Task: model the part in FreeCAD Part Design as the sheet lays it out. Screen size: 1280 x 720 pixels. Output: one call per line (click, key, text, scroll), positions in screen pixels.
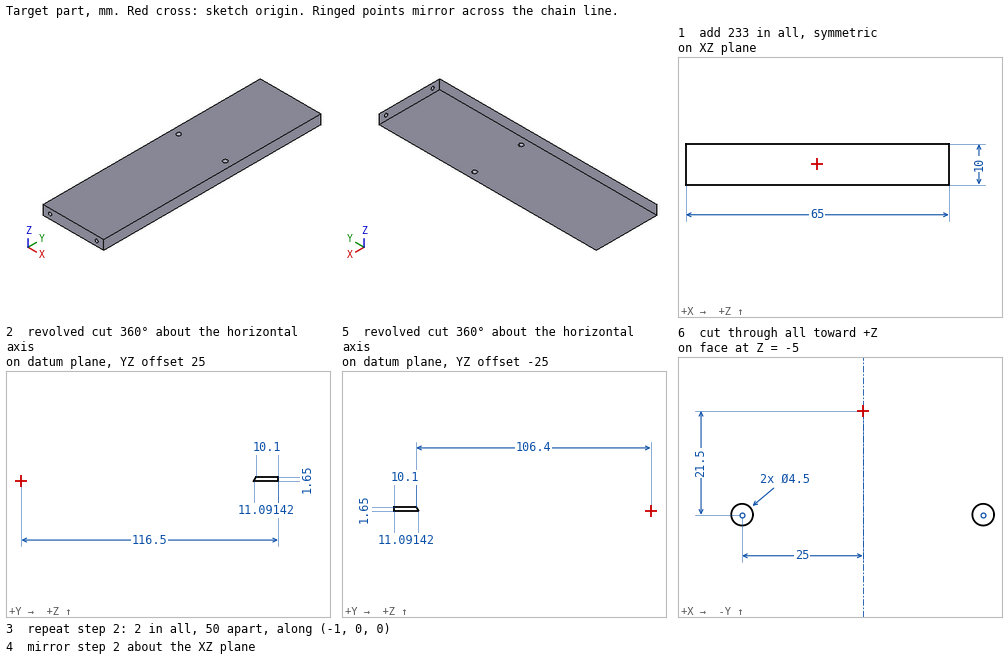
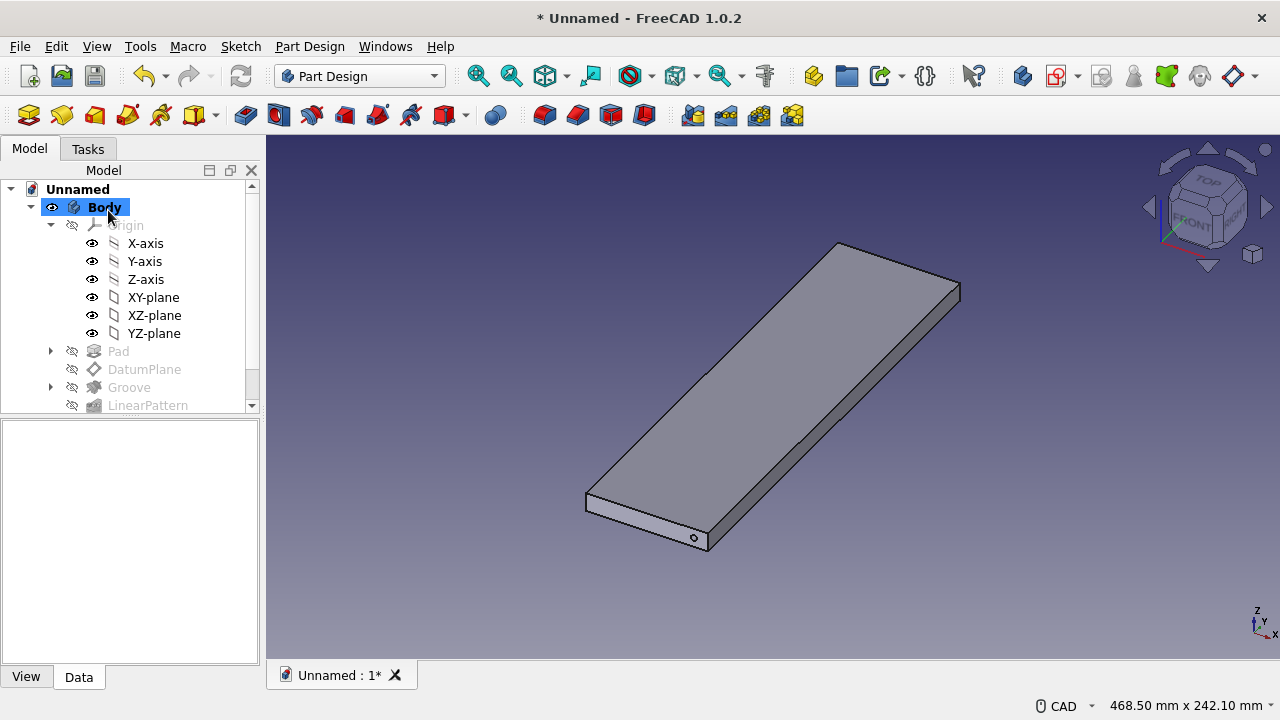
click(137, 333)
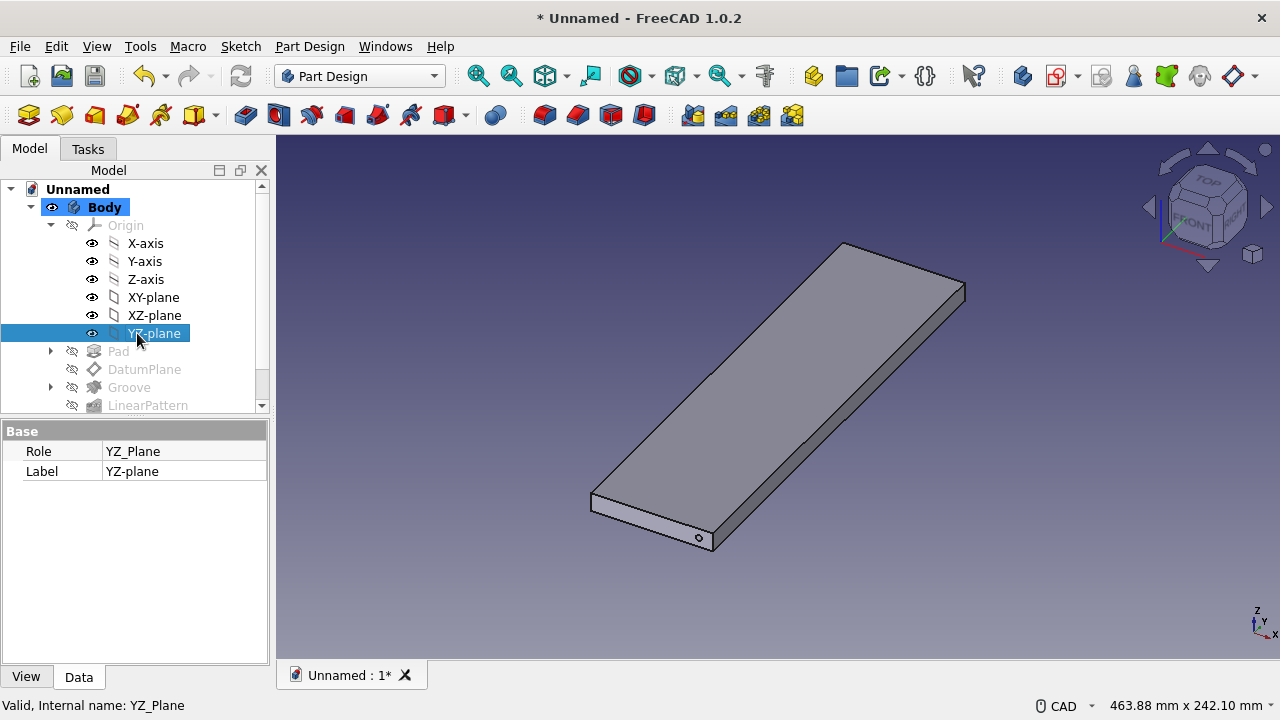
click(1232, 76)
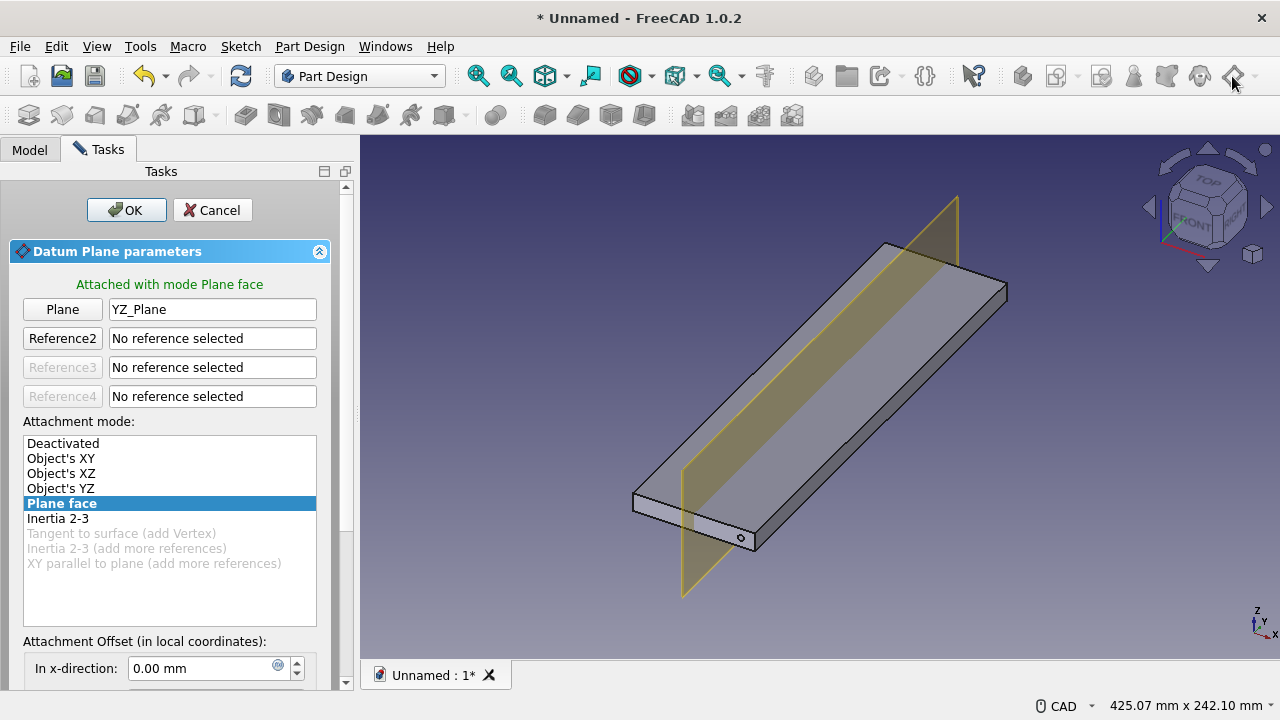
scroll(346, 436, down, 2)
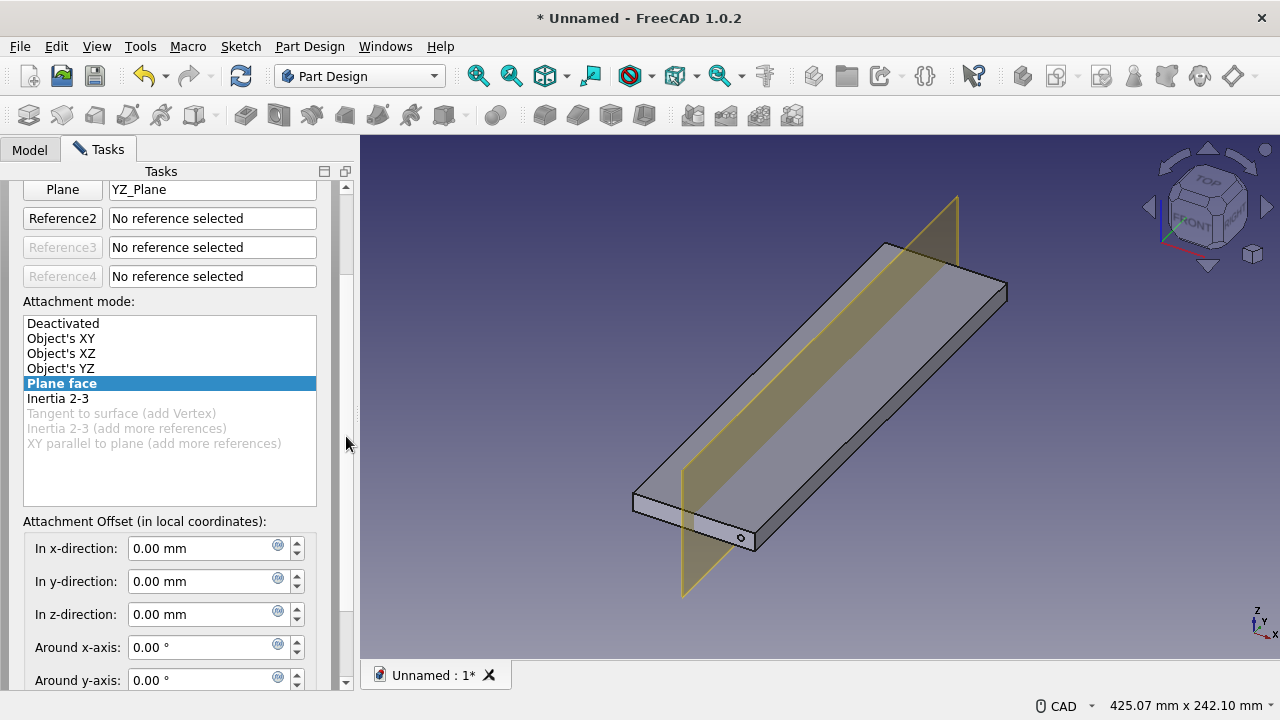
triple_click(210, 614)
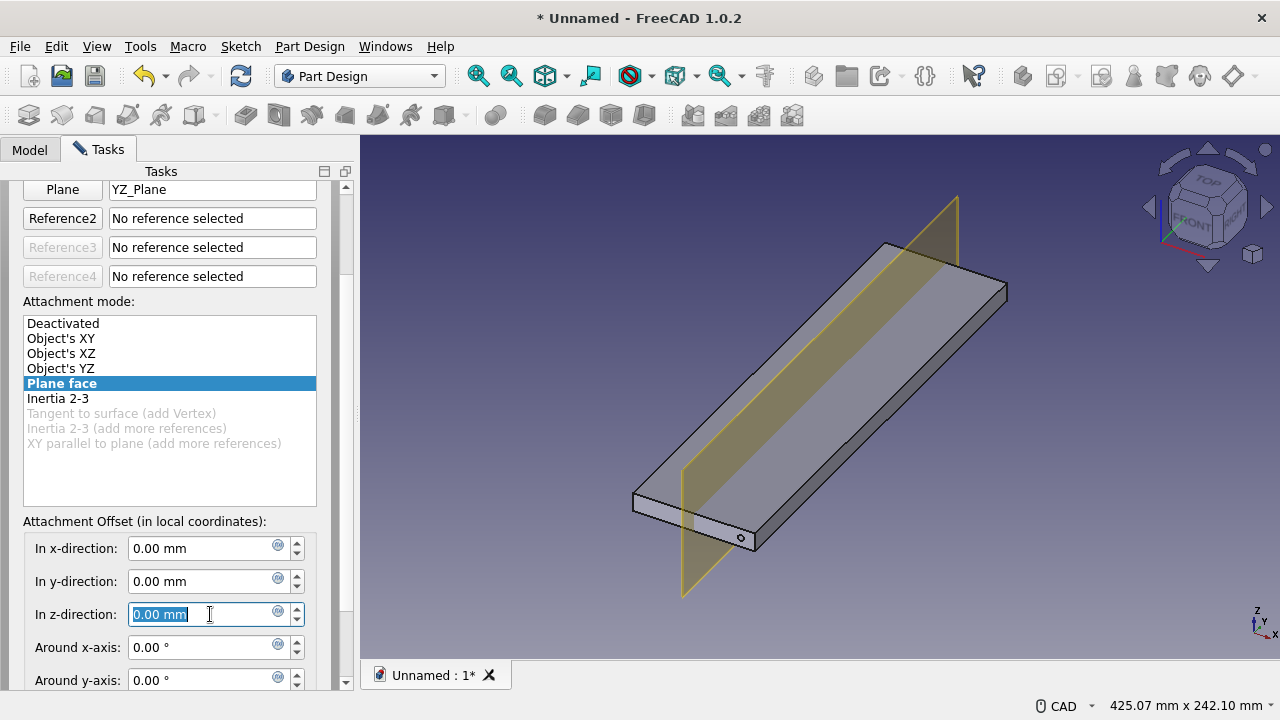
text(-25)
key(Tab)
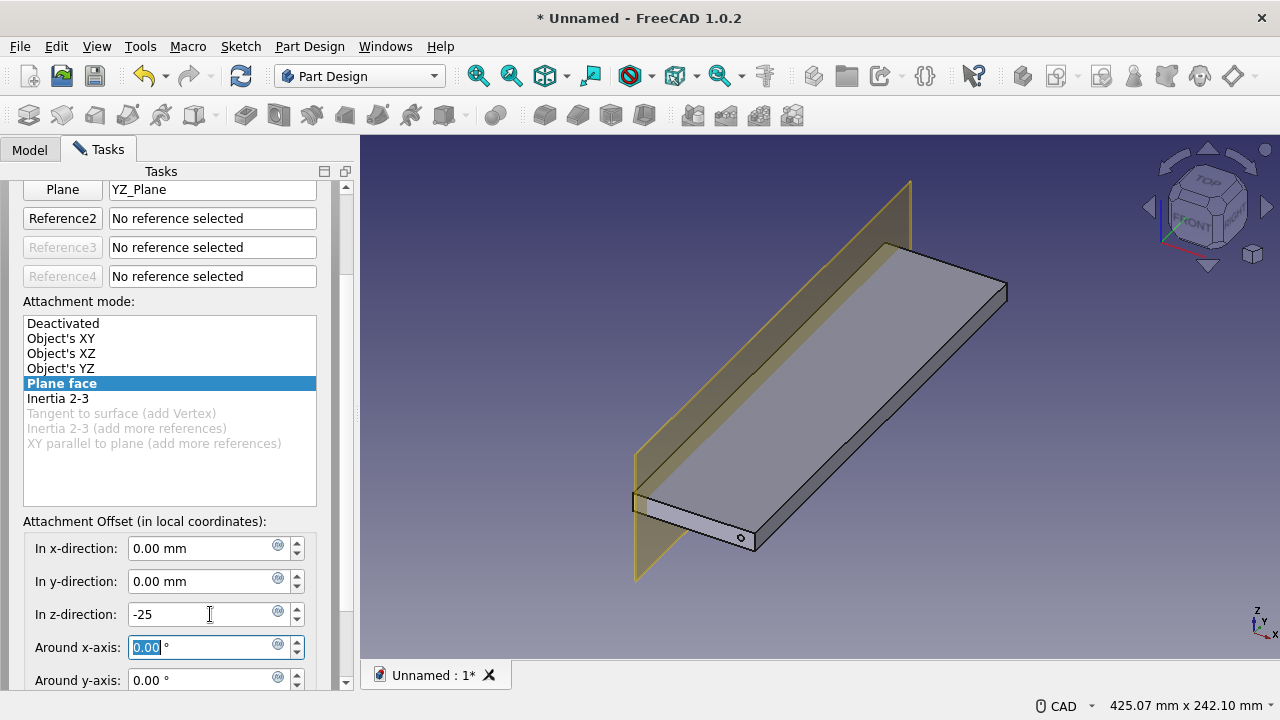
scroll(346, 436, up, 3)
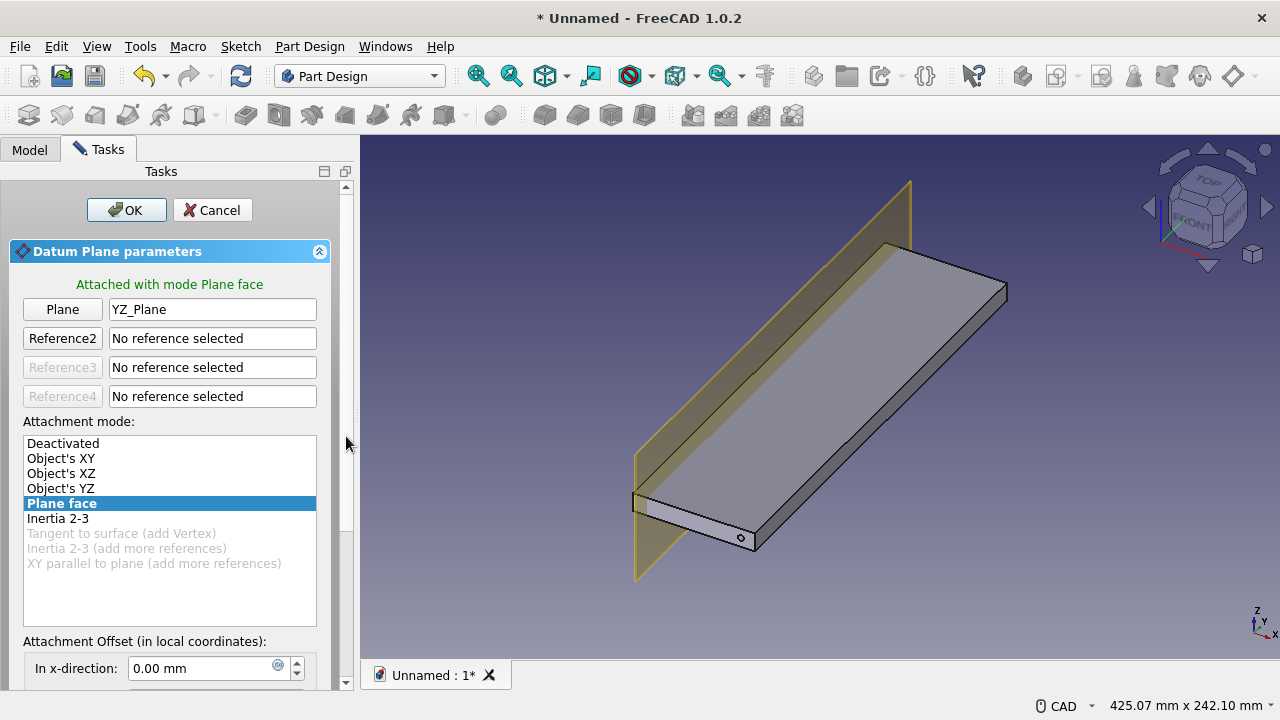
click(127, 210)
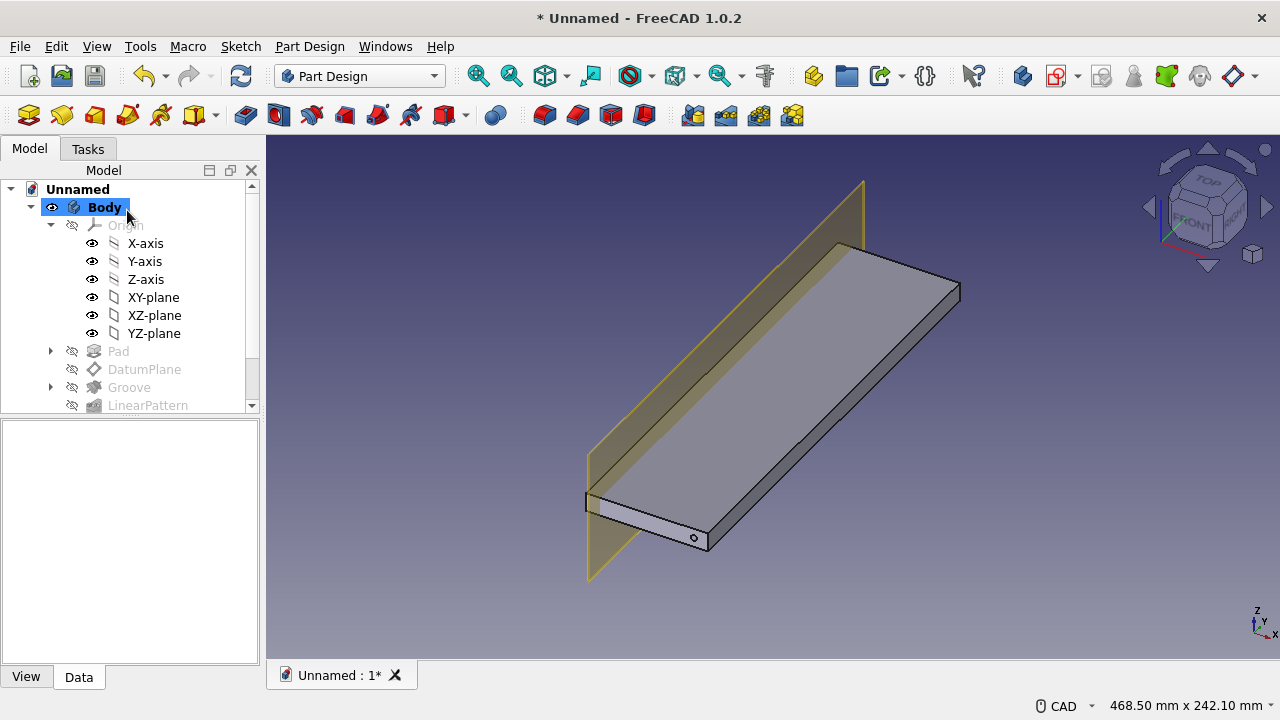
scroll(101, 293, down, 3)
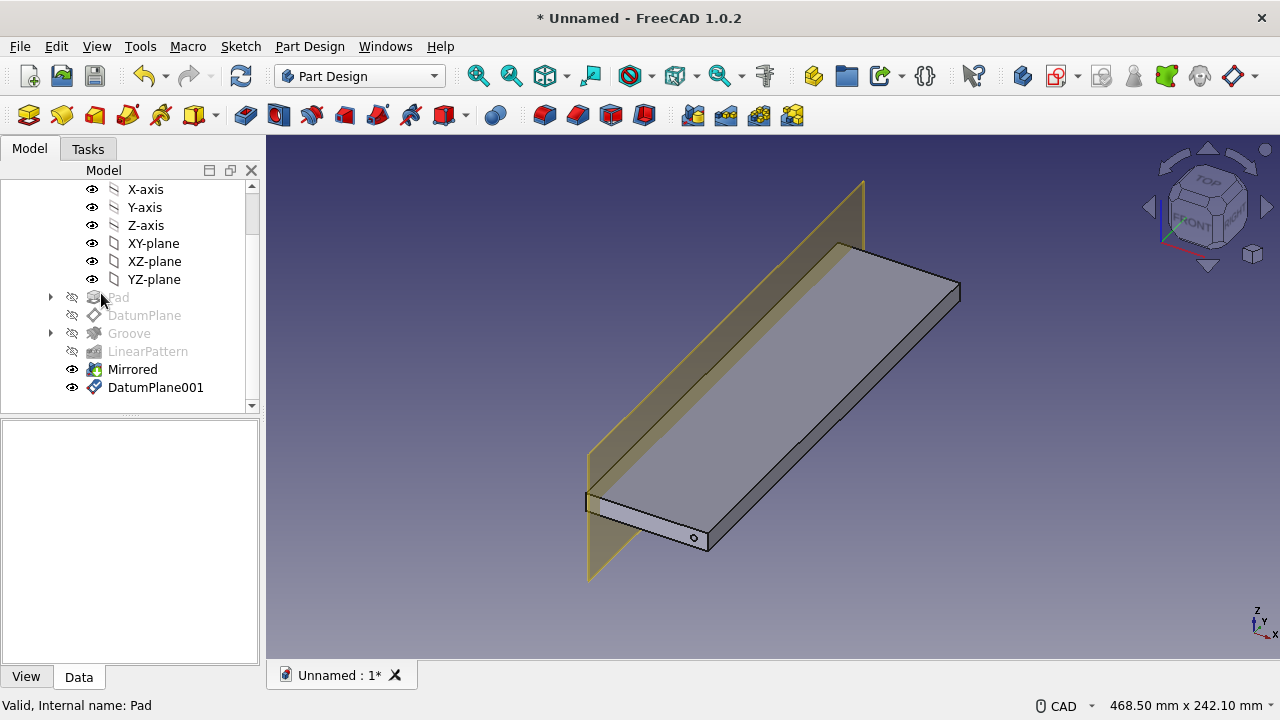
click(117, 387)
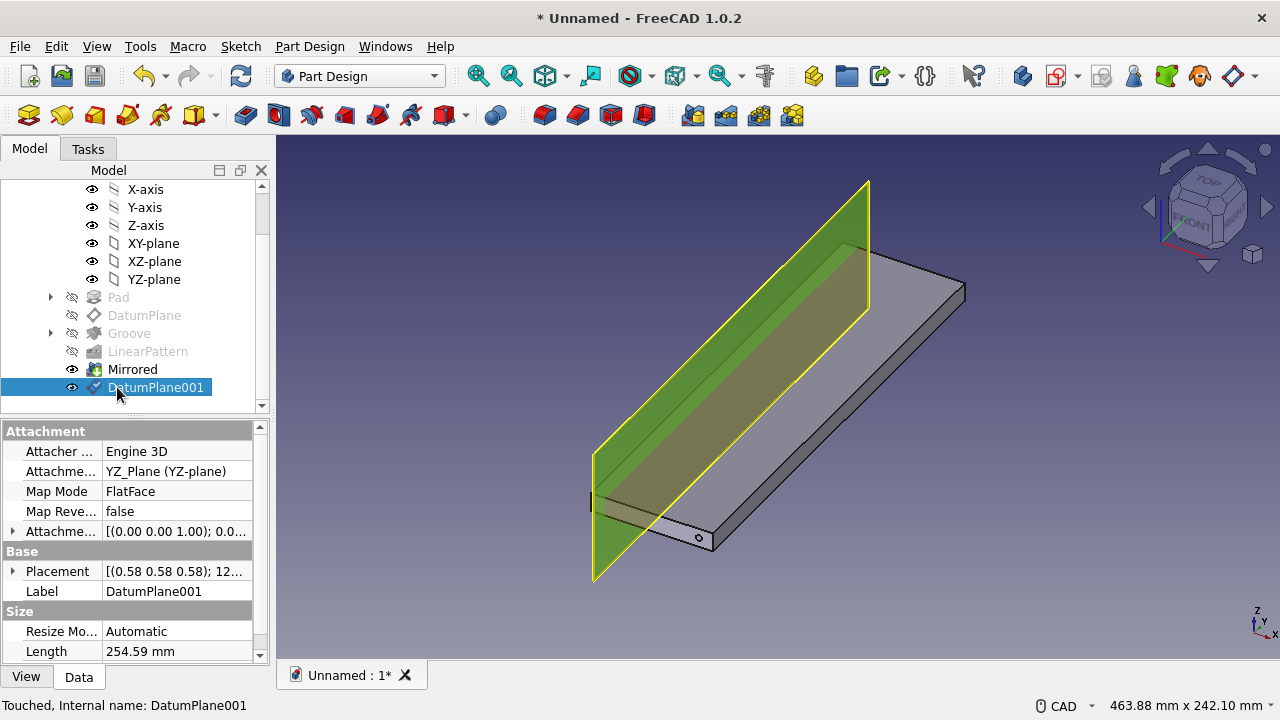
click(1056, 76)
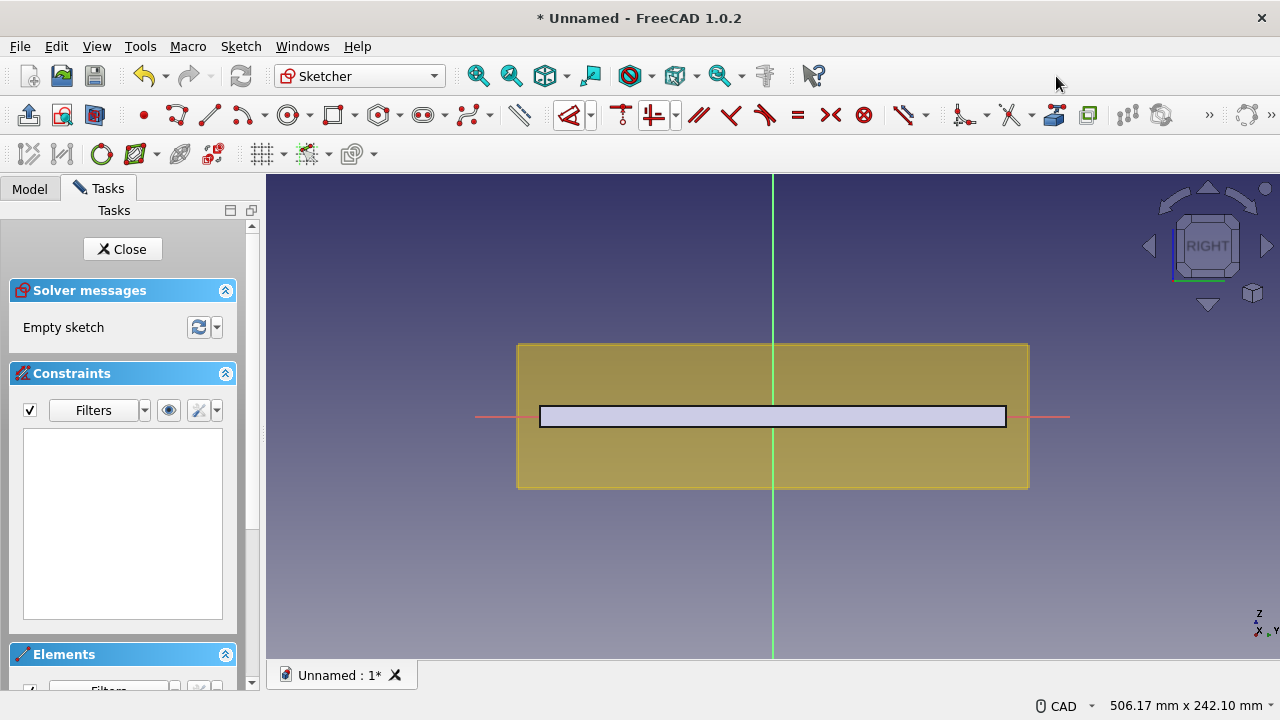
key(q)
key(s)